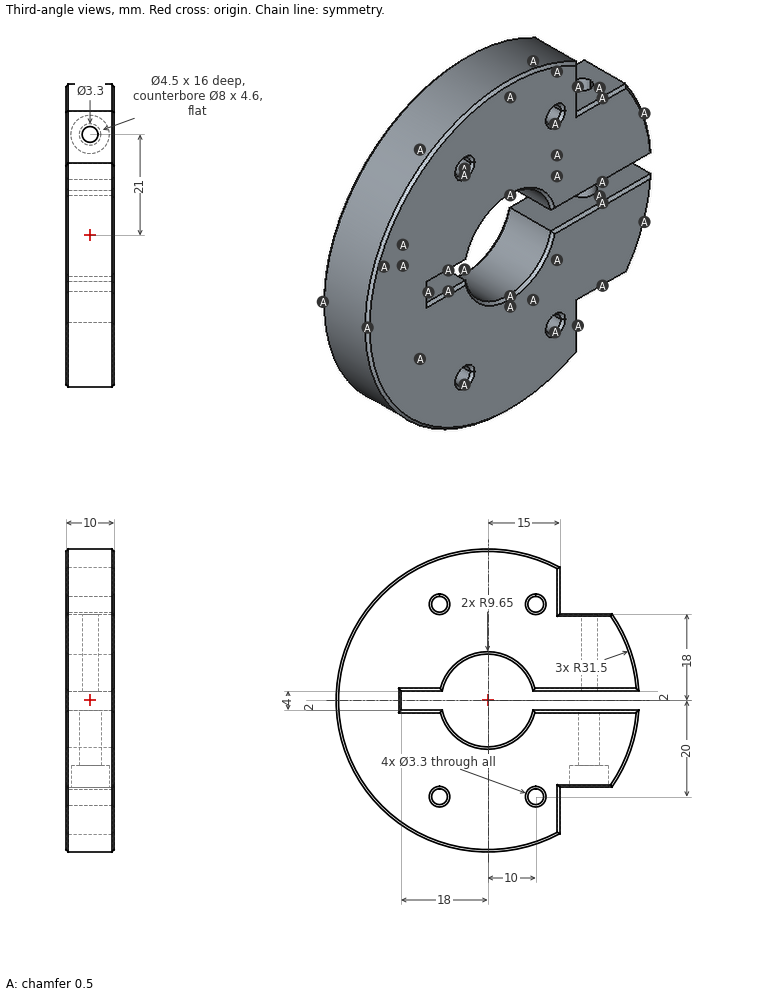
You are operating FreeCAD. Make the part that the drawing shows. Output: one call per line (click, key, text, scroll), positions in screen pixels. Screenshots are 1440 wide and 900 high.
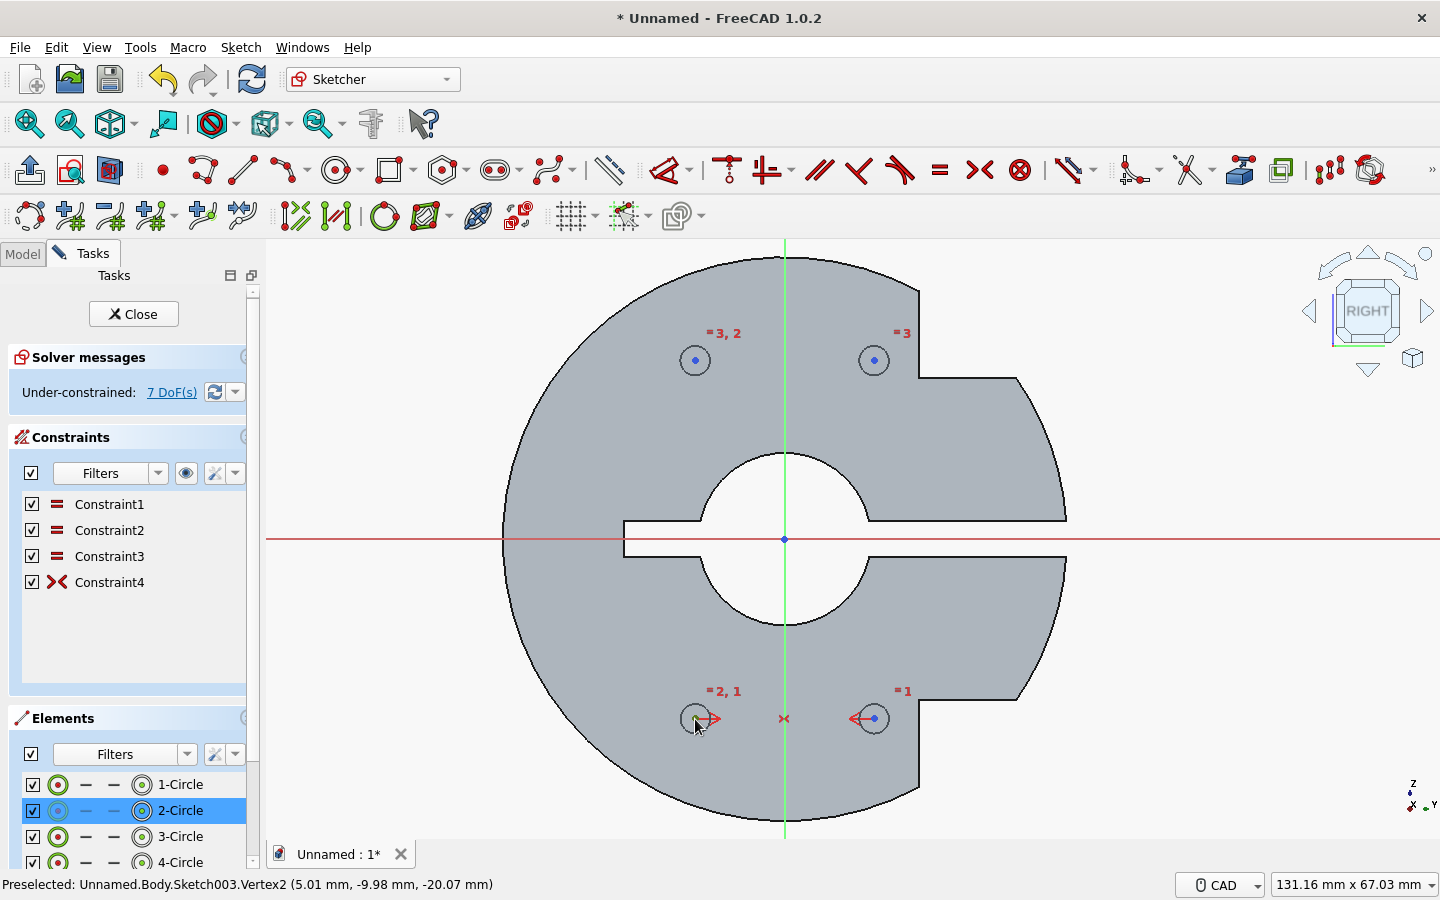
click(695, 361)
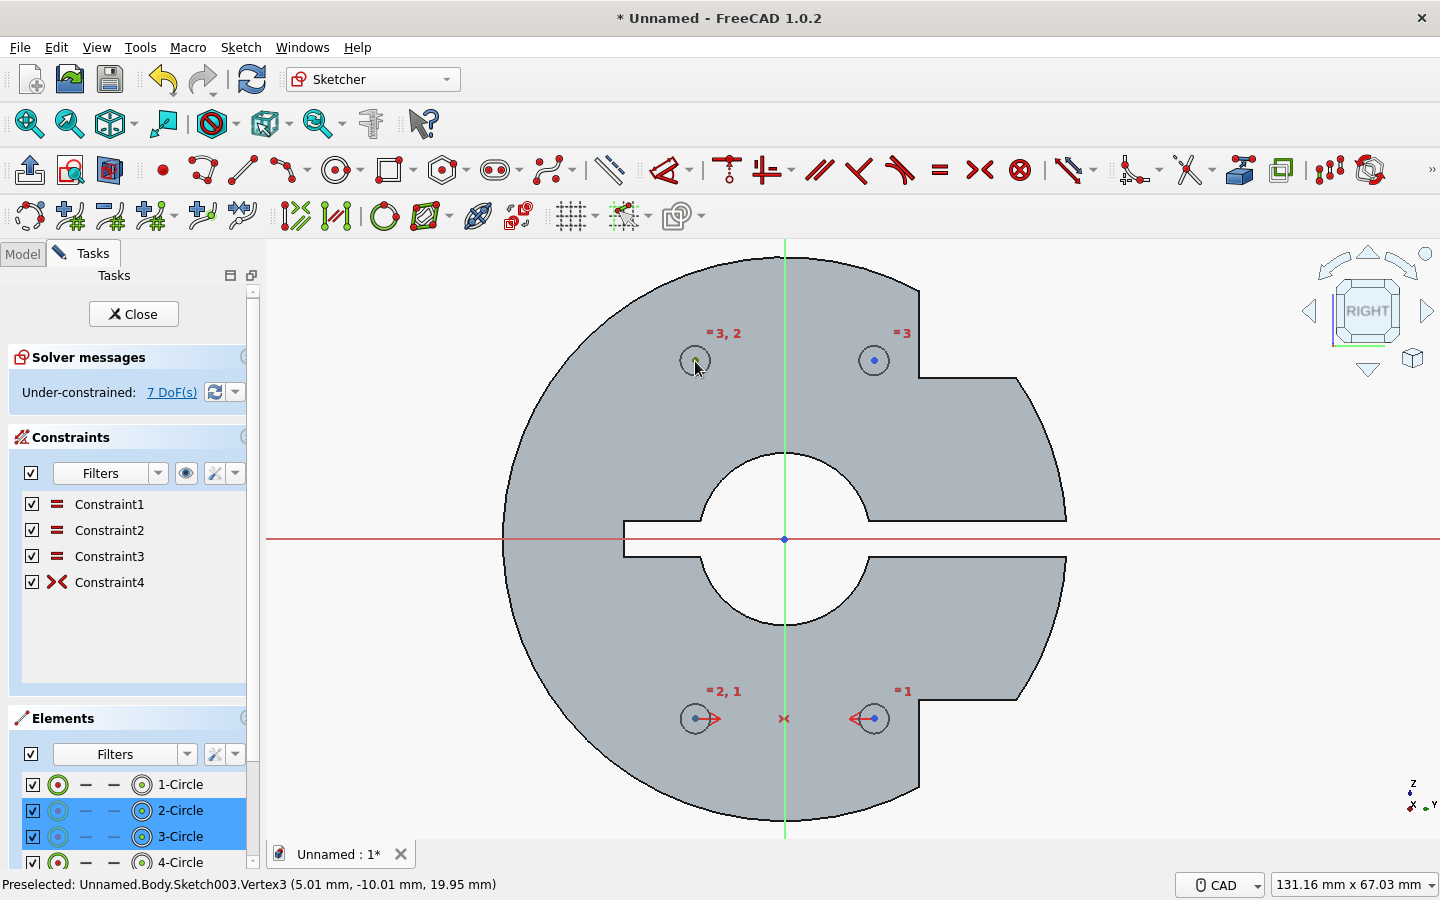
click(364, 539)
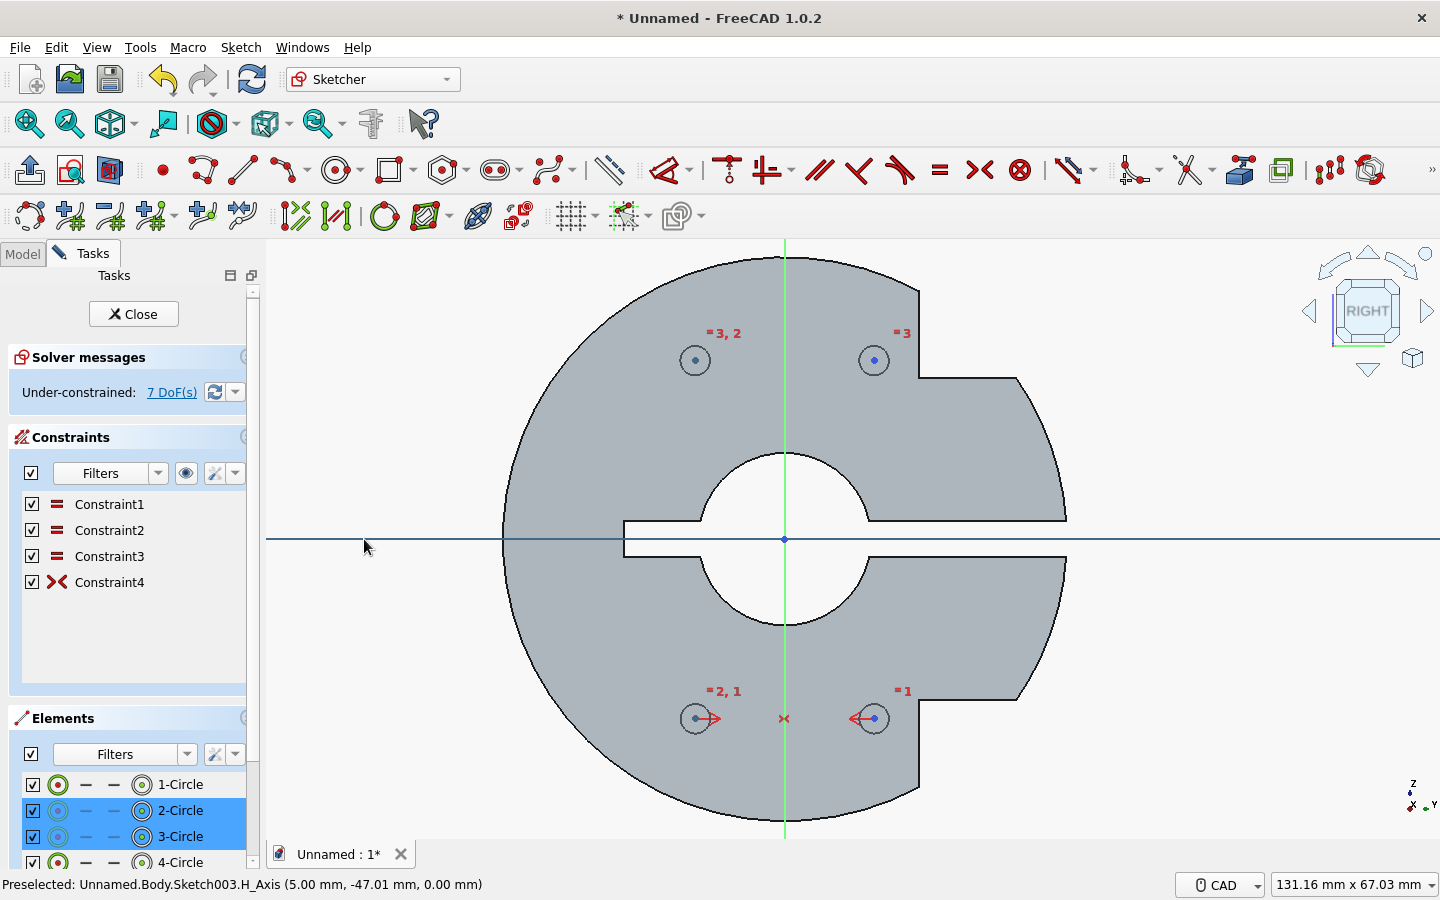
key(s)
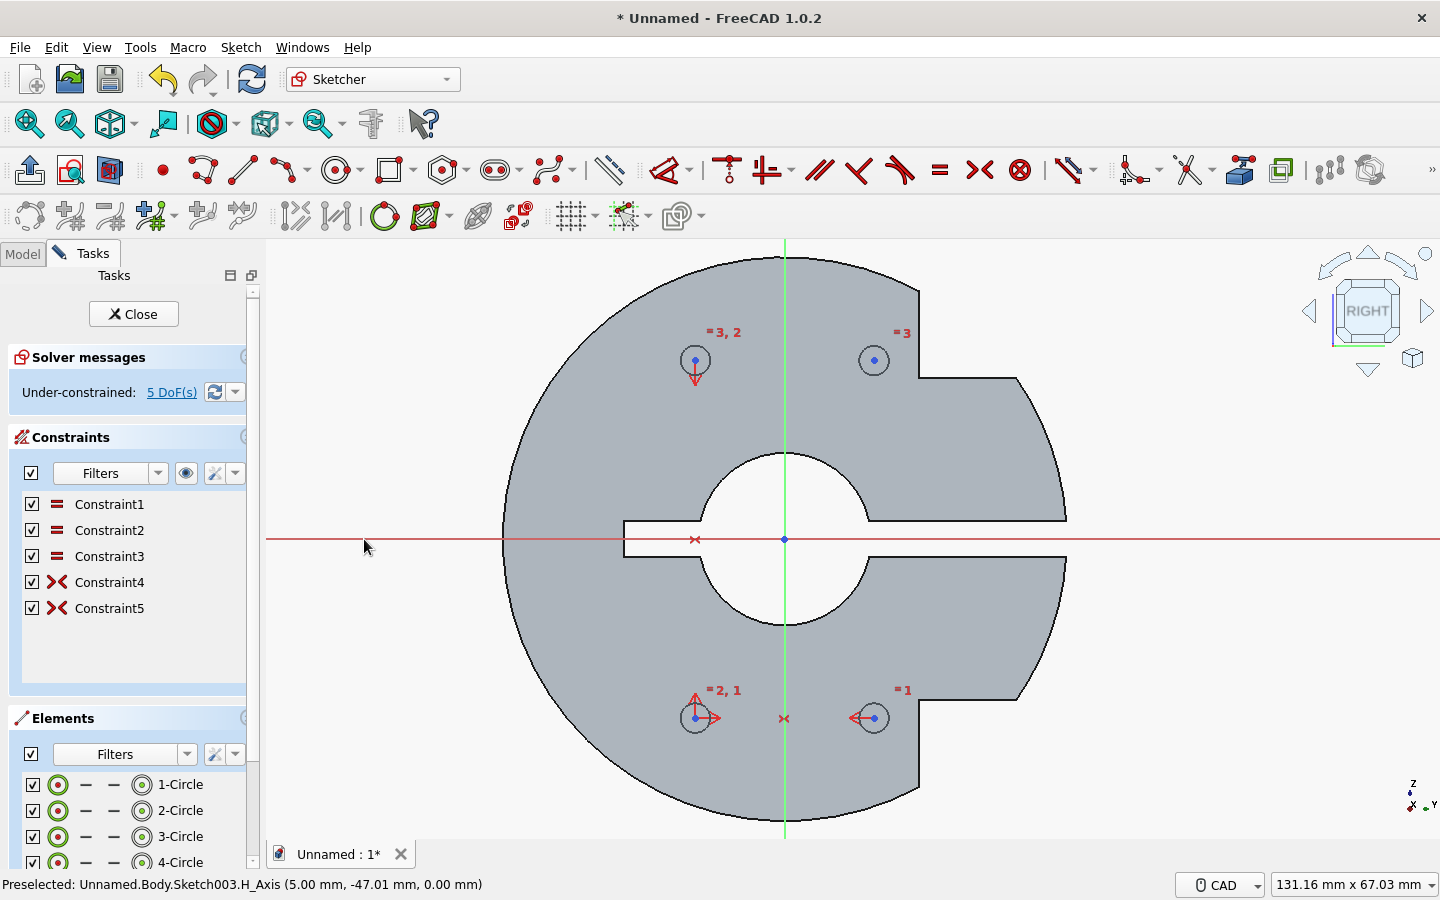
click(874, 718)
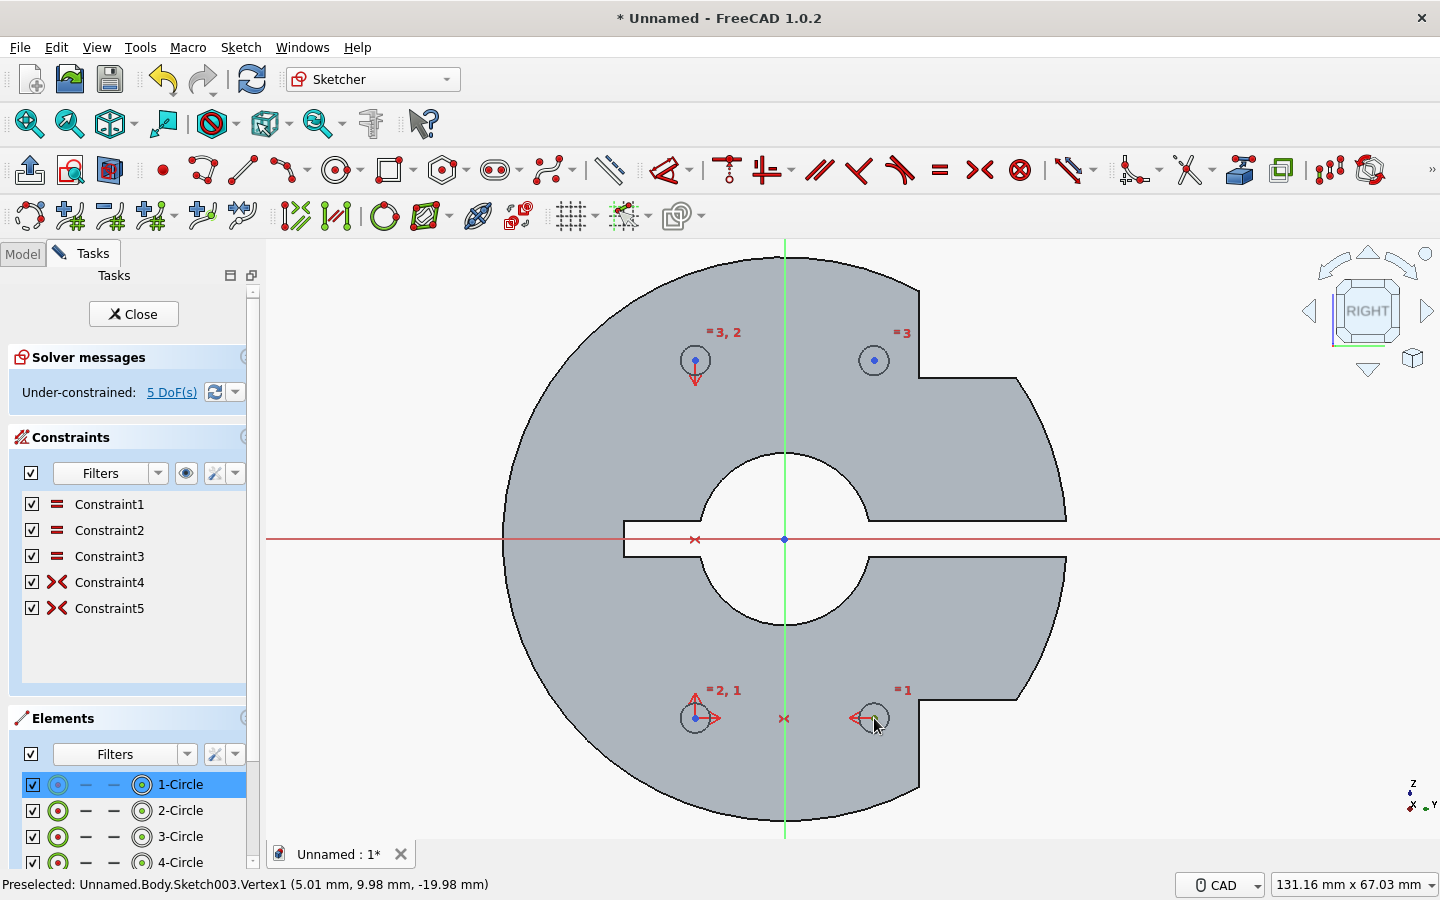
click(874, 361)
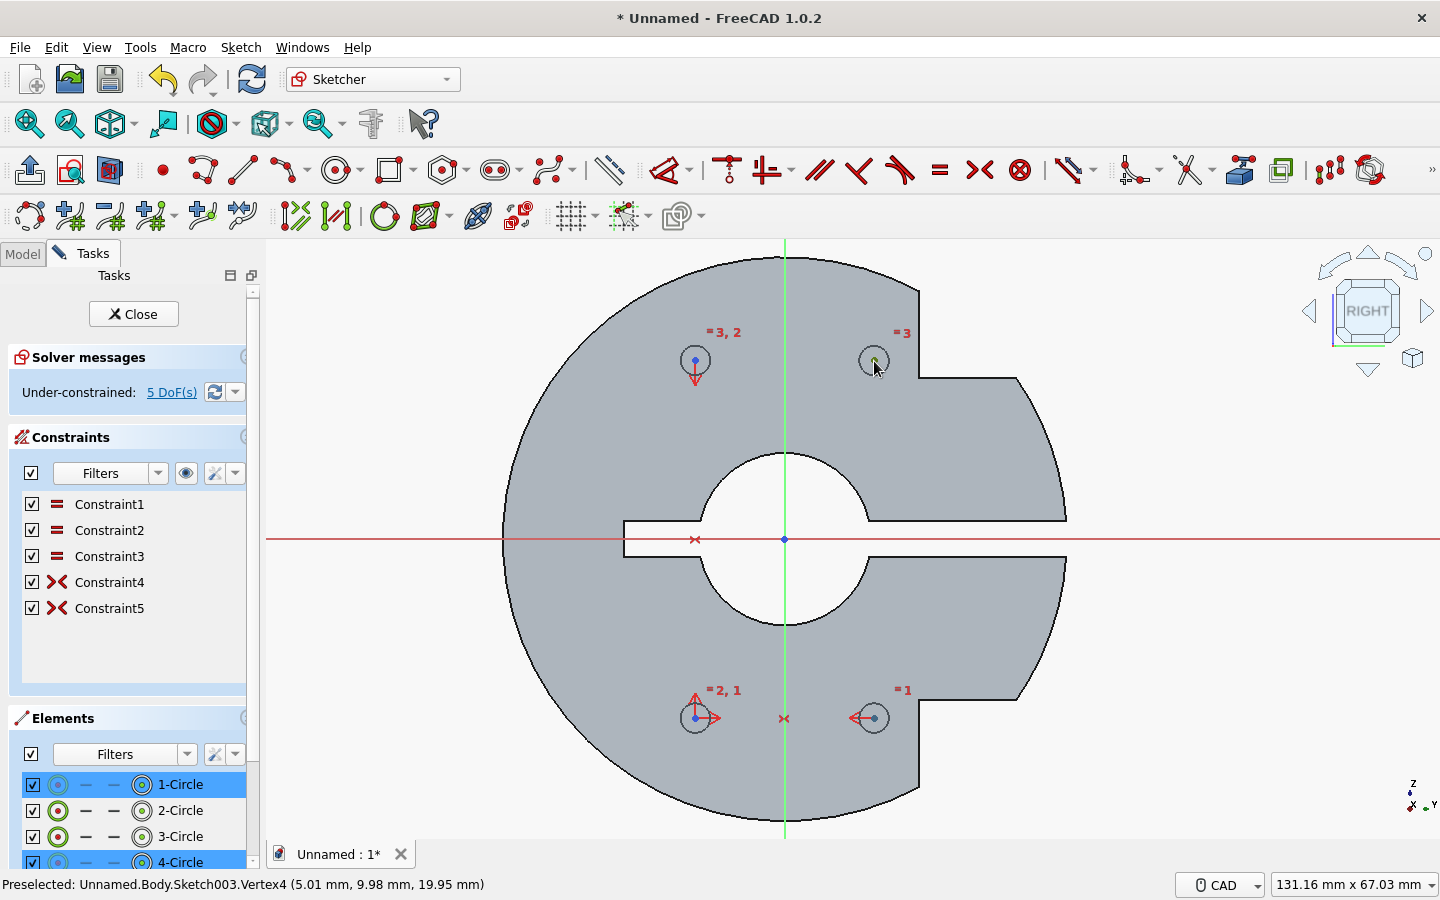
click(364, 539)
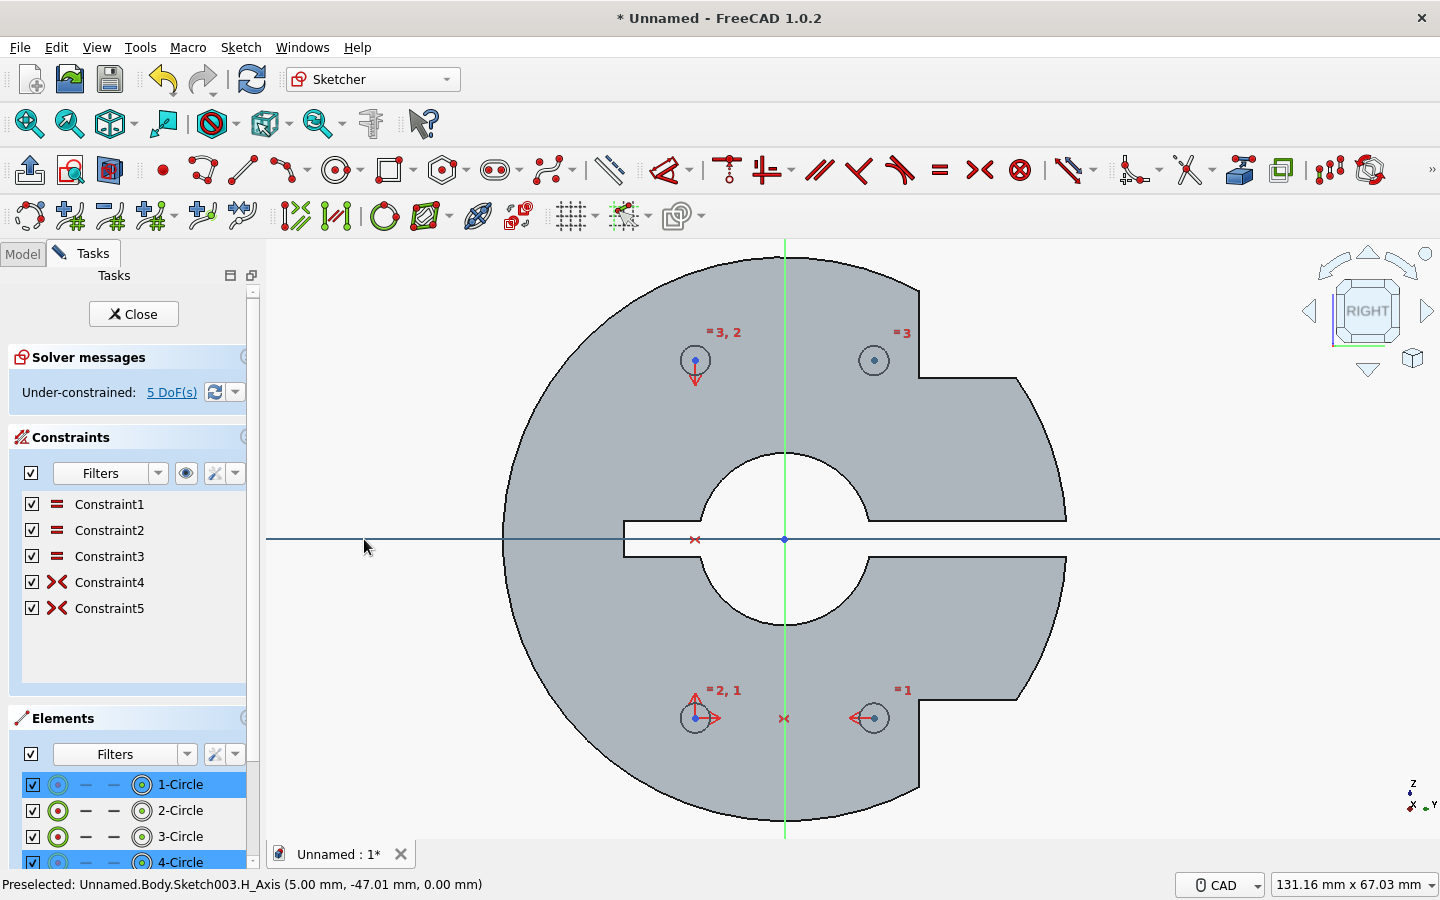
key(s)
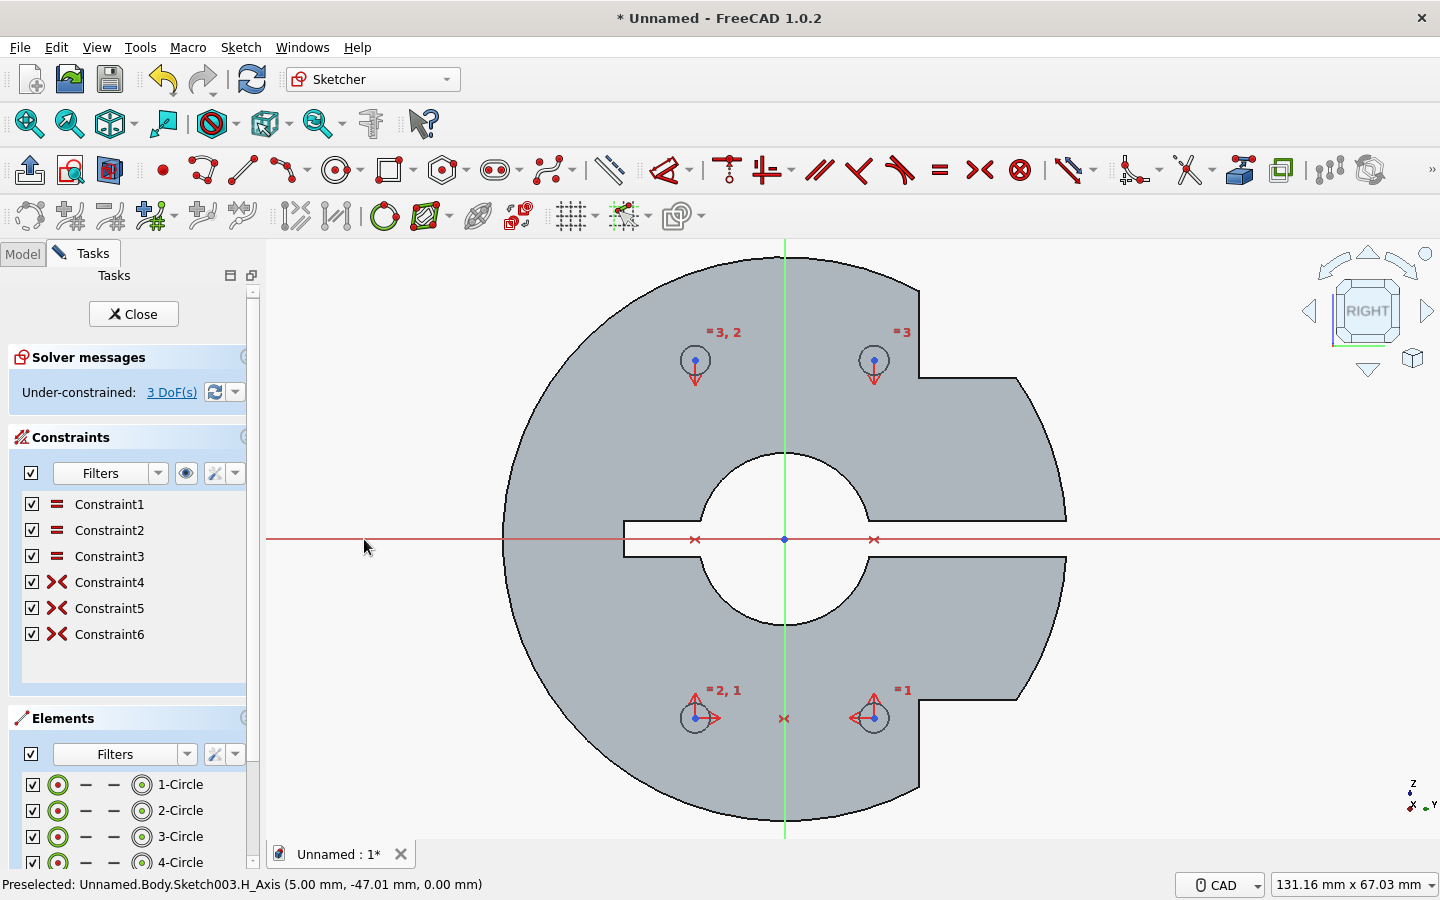
key(d)